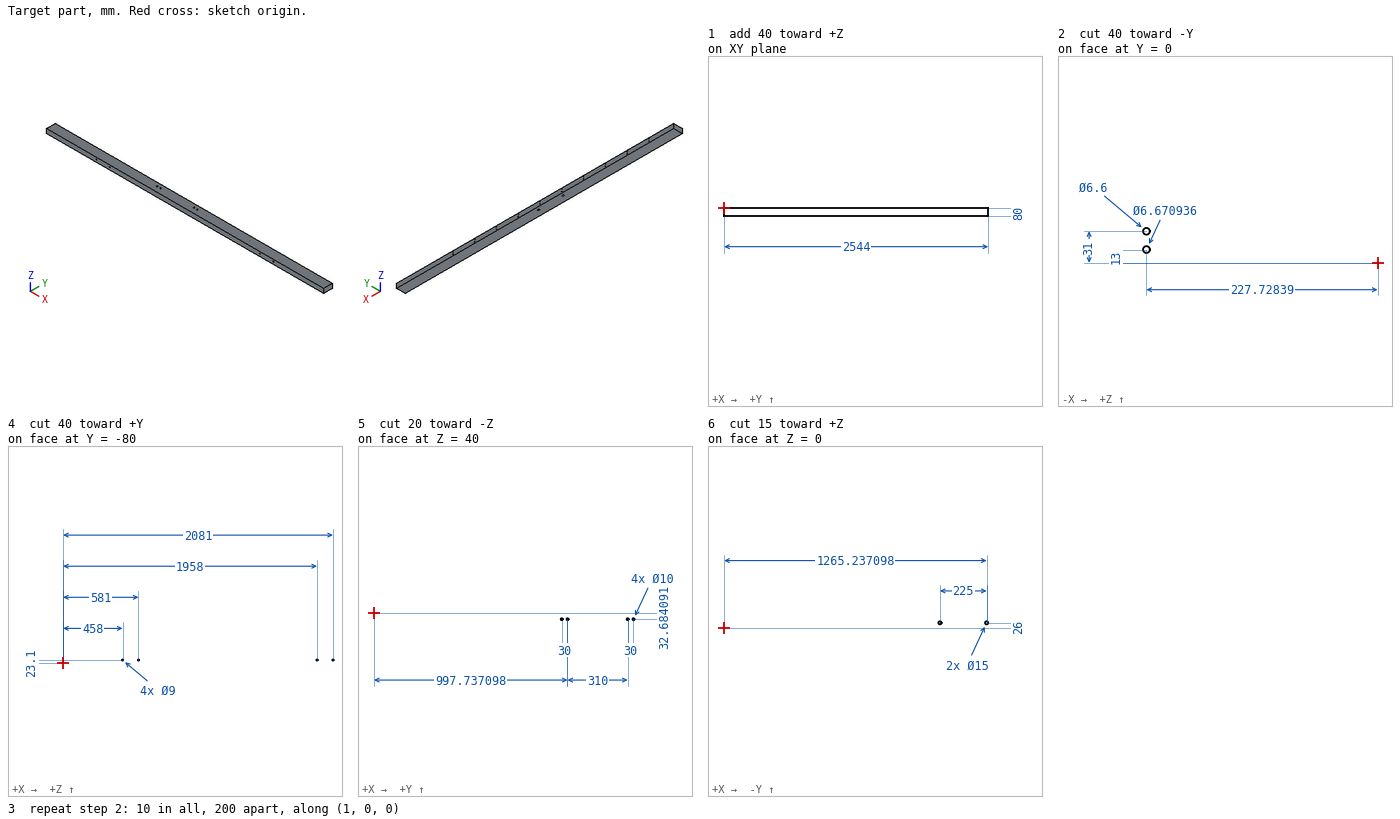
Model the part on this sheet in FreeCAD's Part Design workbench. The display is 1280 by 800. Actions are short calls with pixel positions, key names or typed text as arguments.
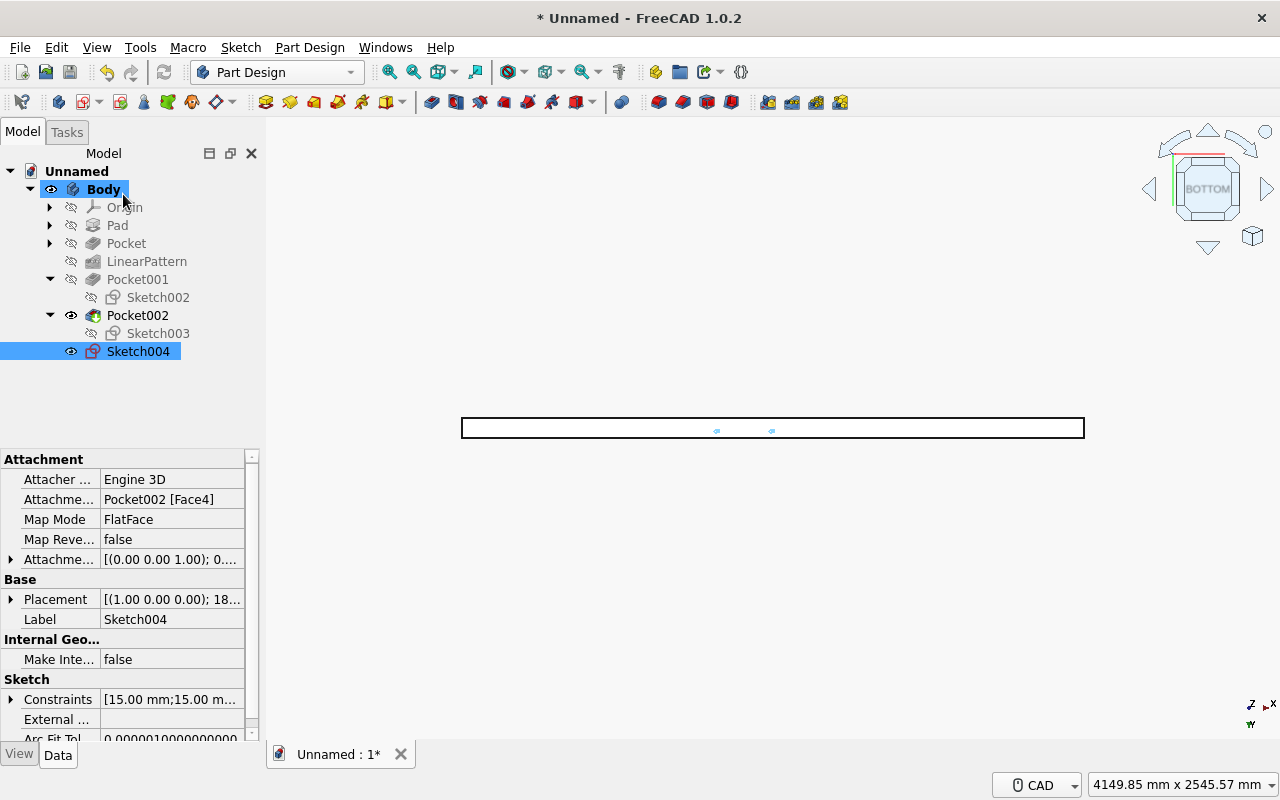
click(432, 102)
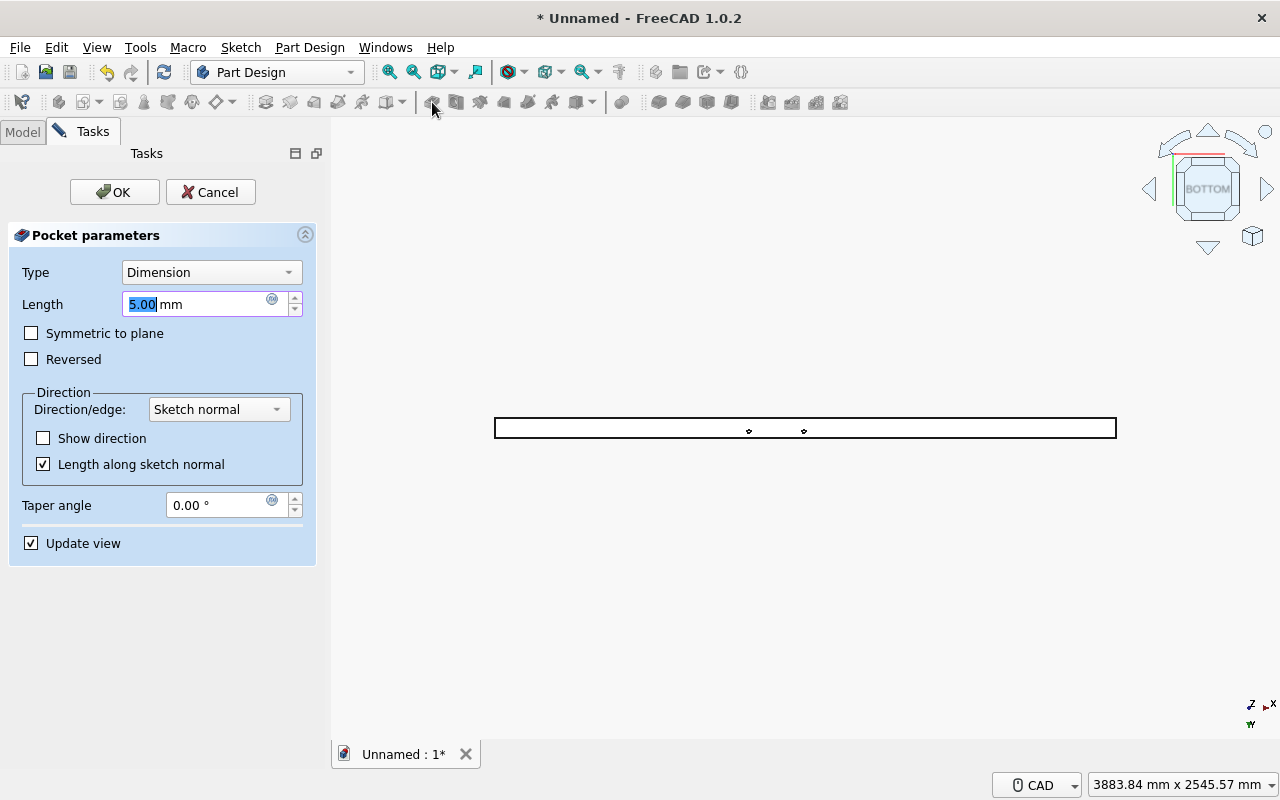
text(15)
key(Tab)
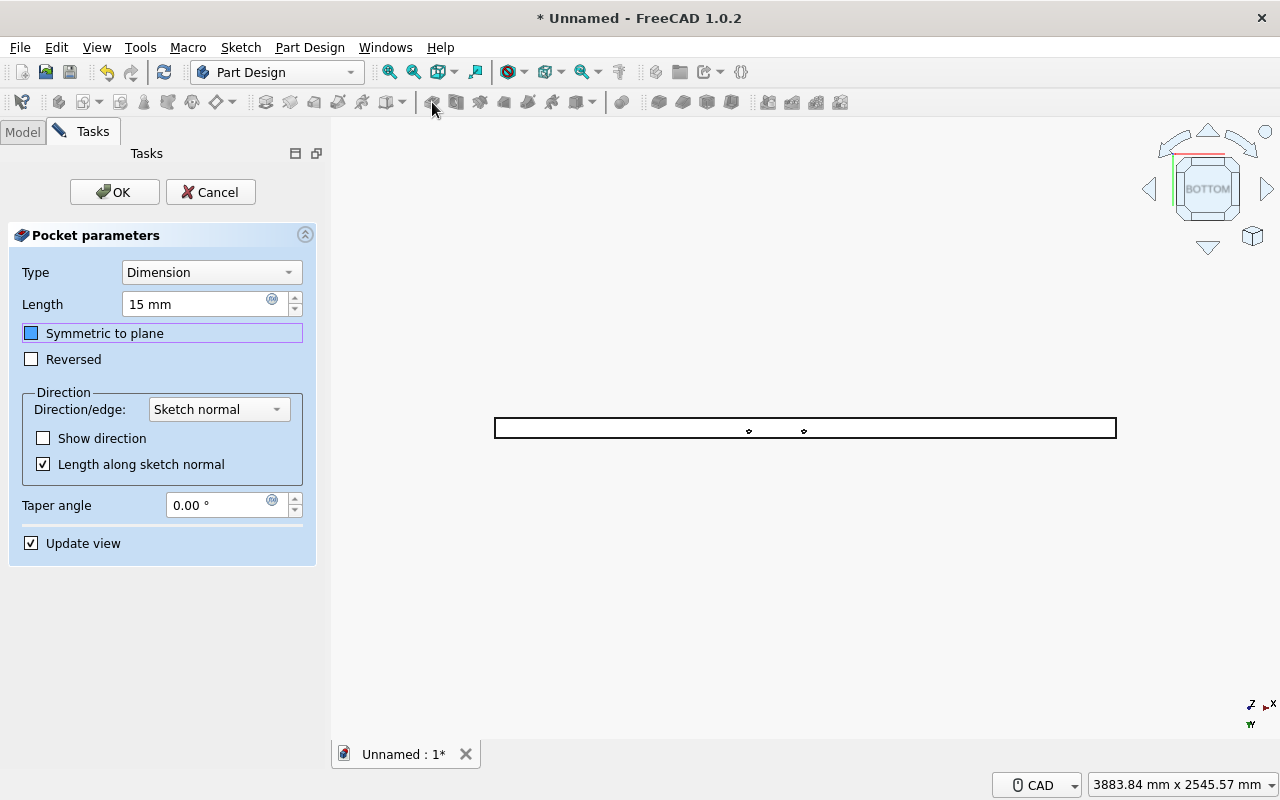
click(115, 192)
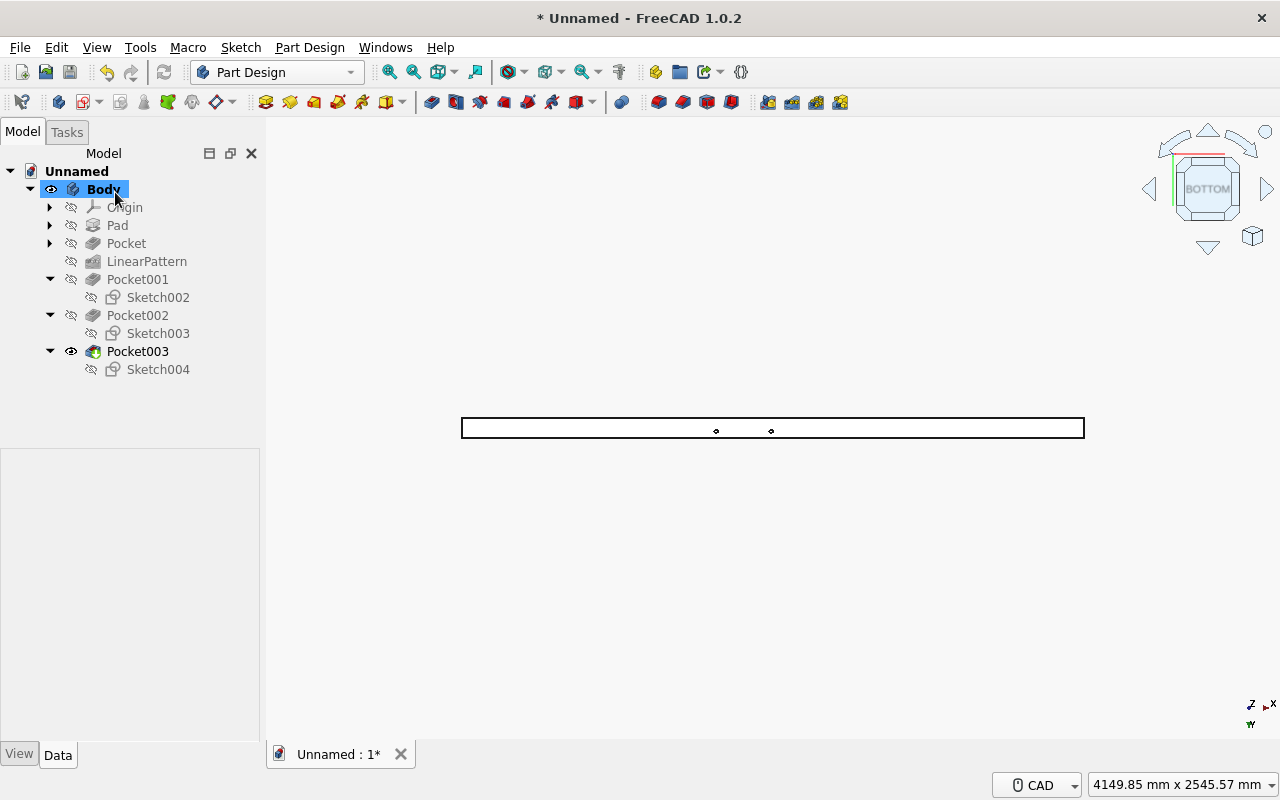
key(0)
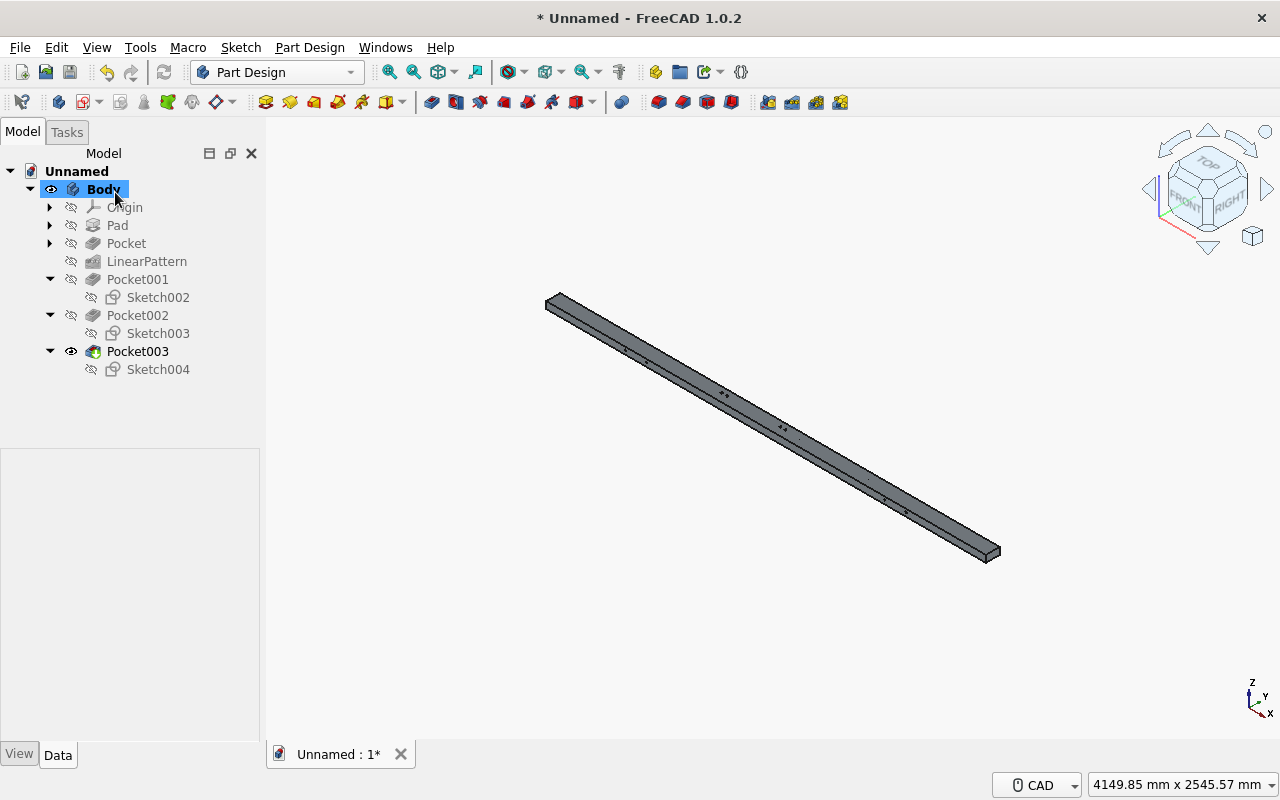
key(v)
key(f)